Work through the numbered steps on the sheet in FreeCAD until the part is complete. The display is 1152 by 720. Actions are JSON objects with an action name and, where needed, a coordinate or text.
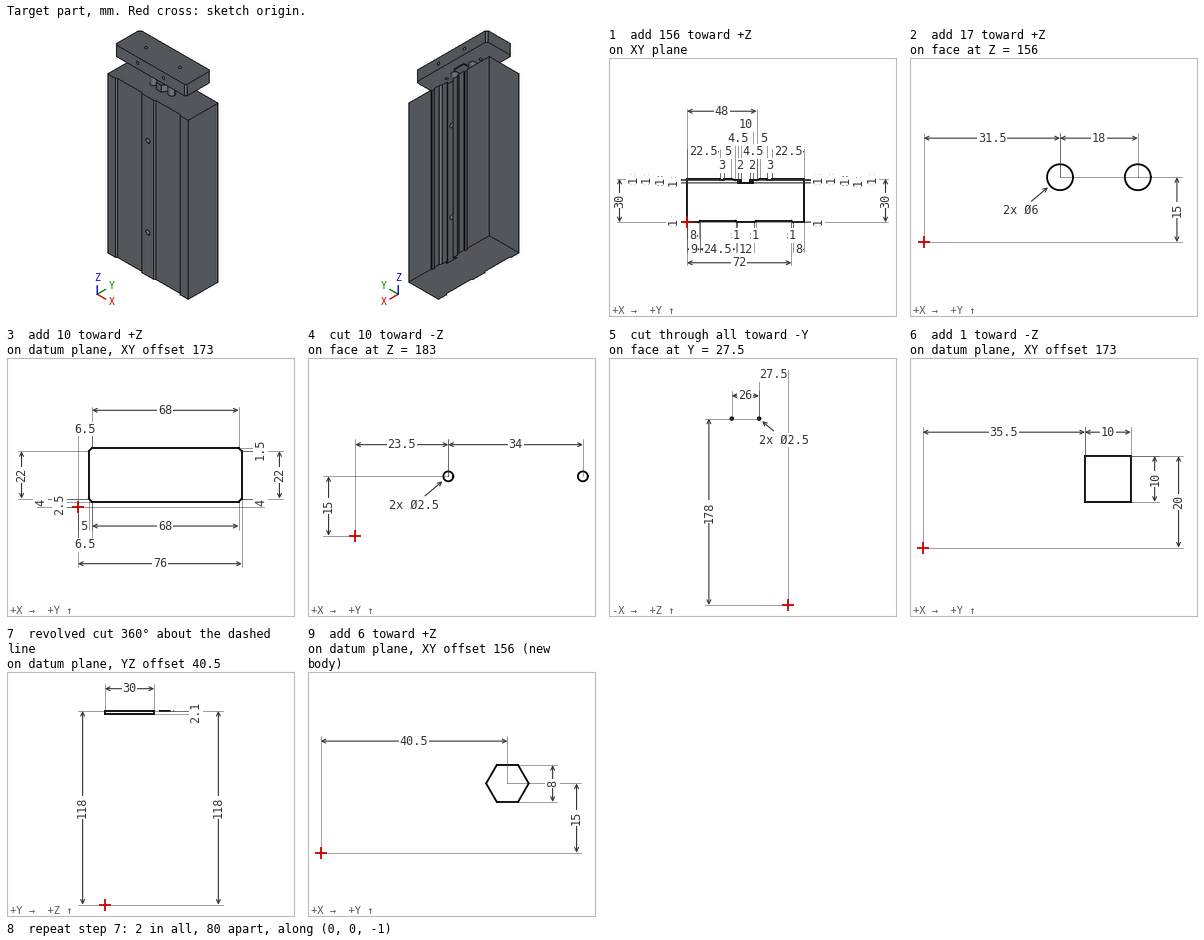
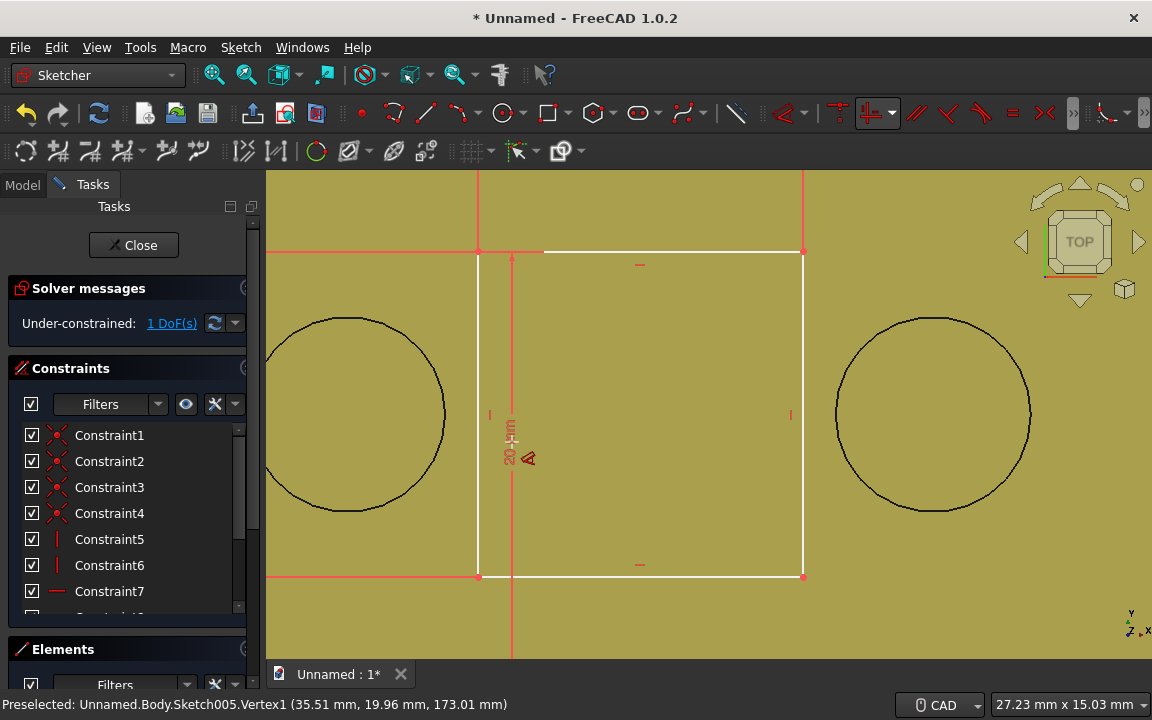
{"action": "left_click", "coordinate": [478, 252]}
{"action": "left_click", "coordinate": [386, 218]}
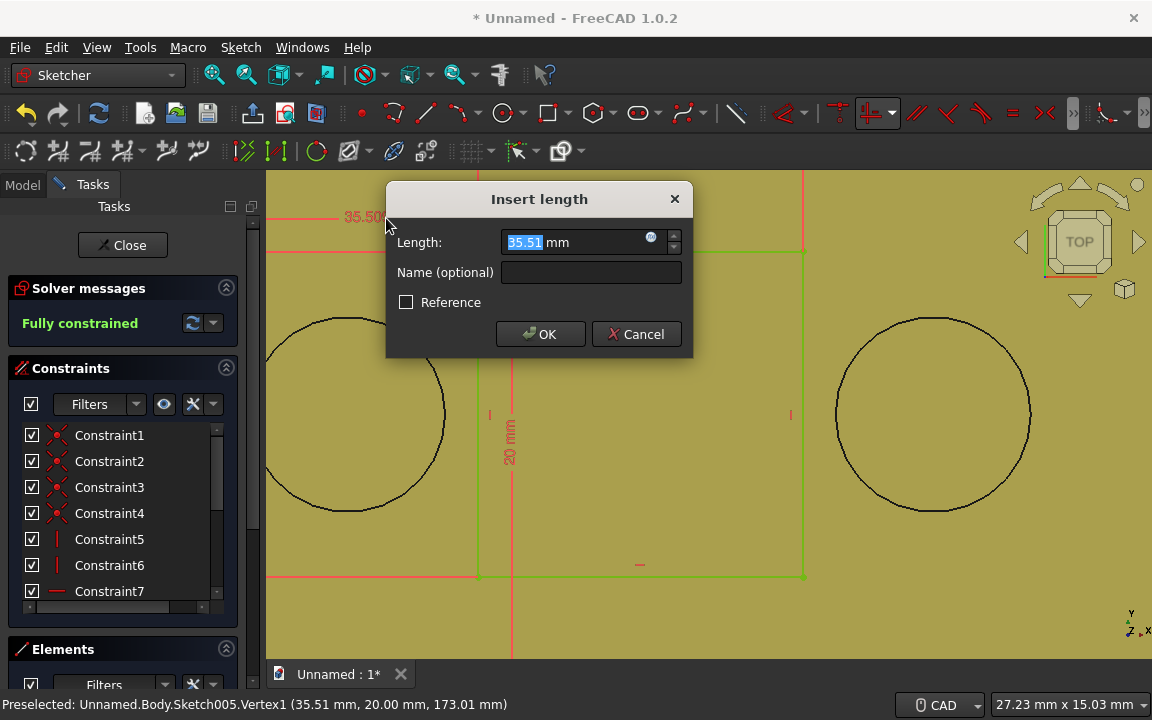
{"action": "type", "text": "35.5"}
{"action": "key", "text": "Return"}
{"action": "key", "text": "Escape"}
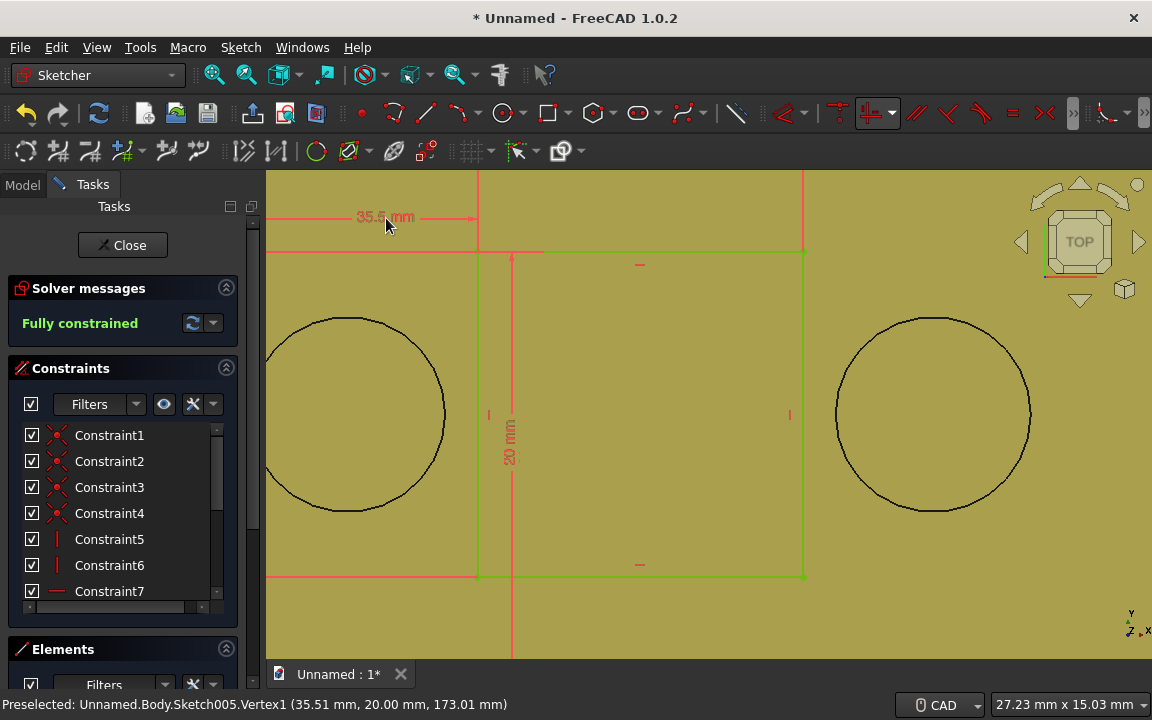
{"action": "left_click", "coordinate": [123, 245]}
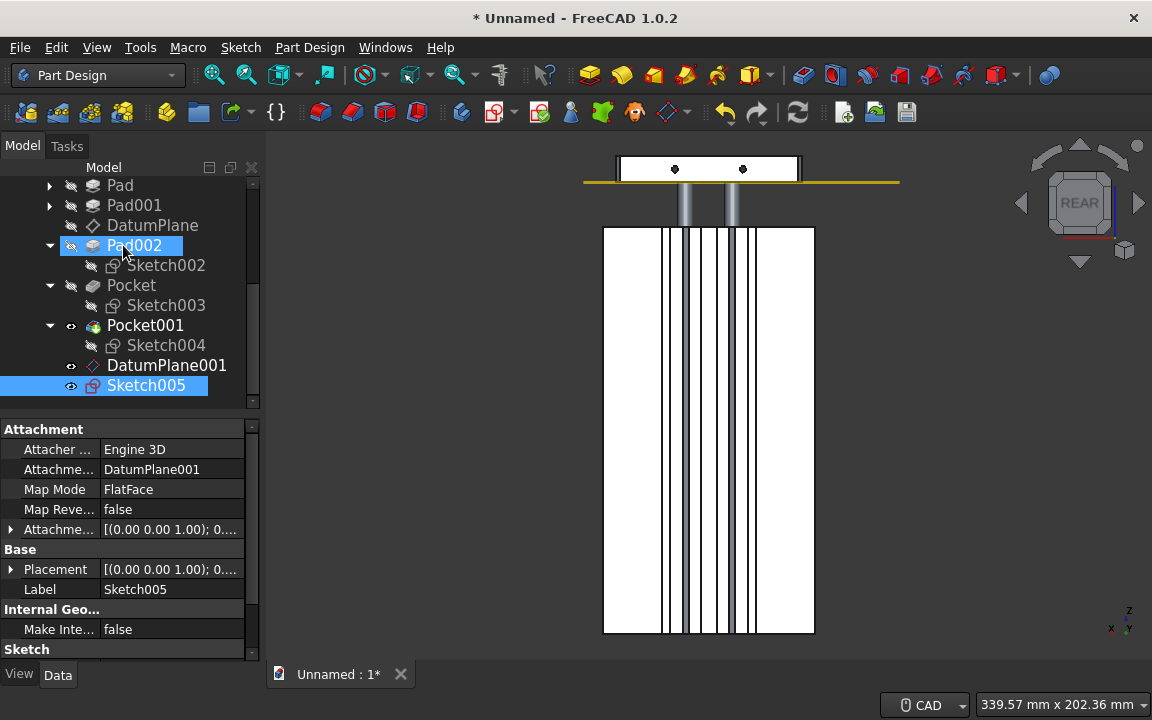
{"action": "left_click", "coordinate": [590, 76]}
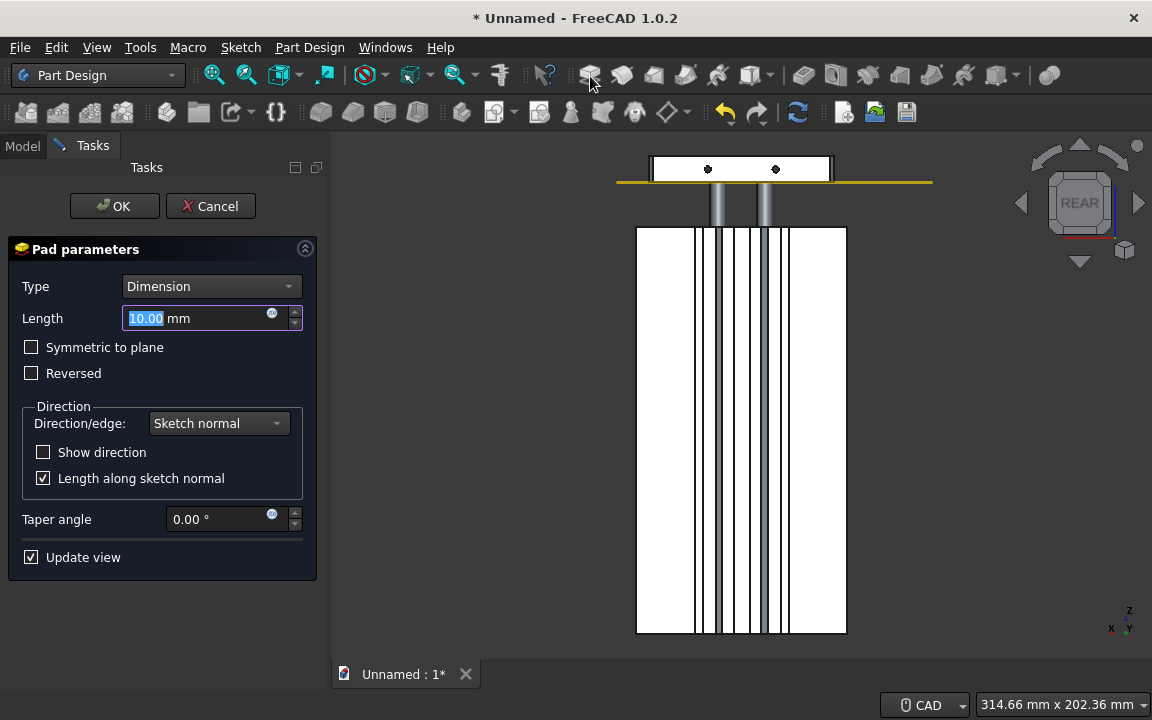
{"action": "type", "text": "1"}
{"action": "key", "text": "Tab"}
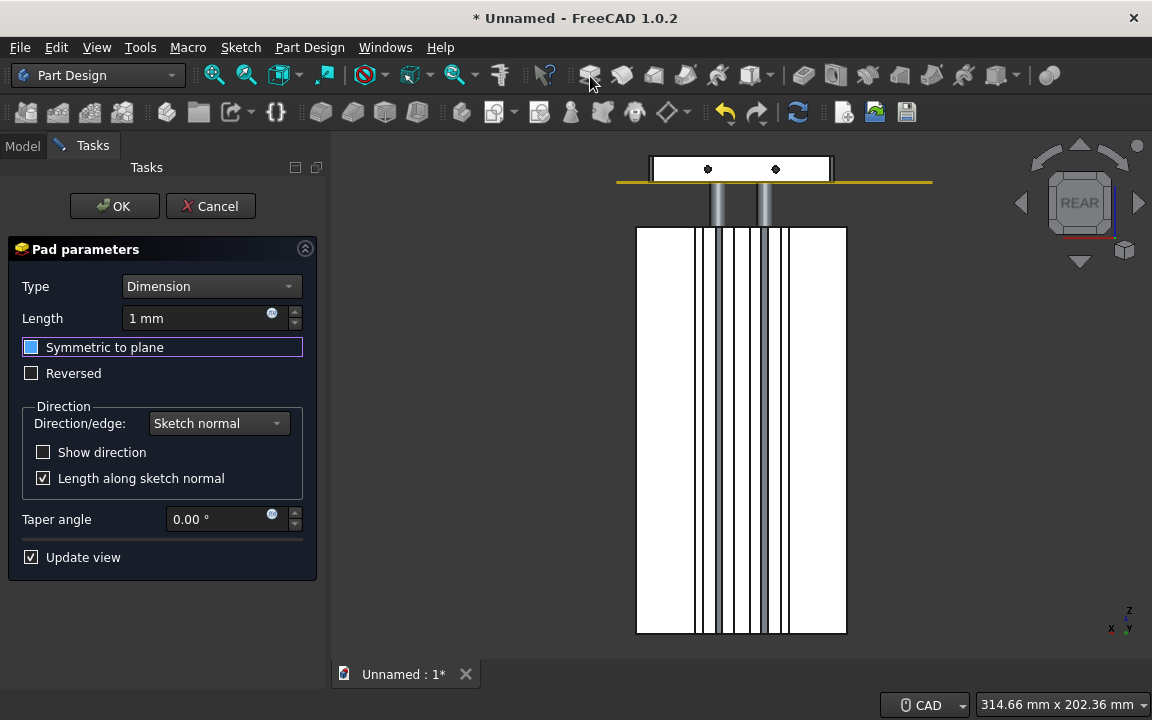
{"action": "left_click", "coordinate": [30, 373]}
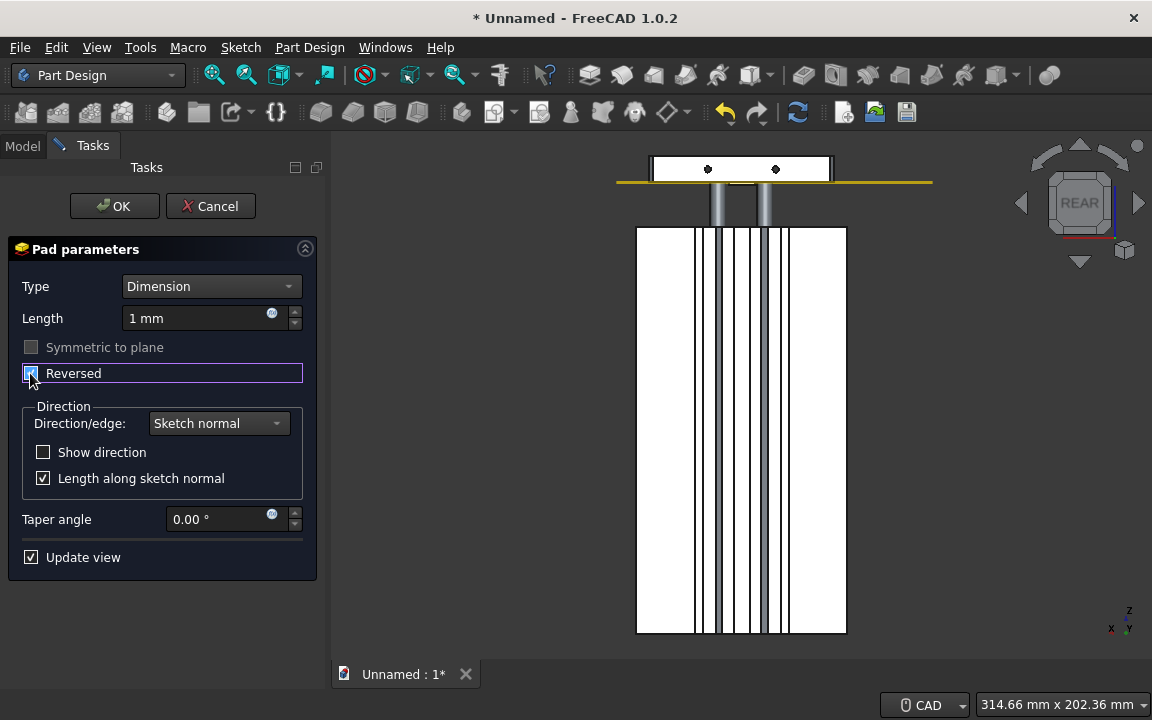
{"action": "left_click", "coordinate": [115, 206]}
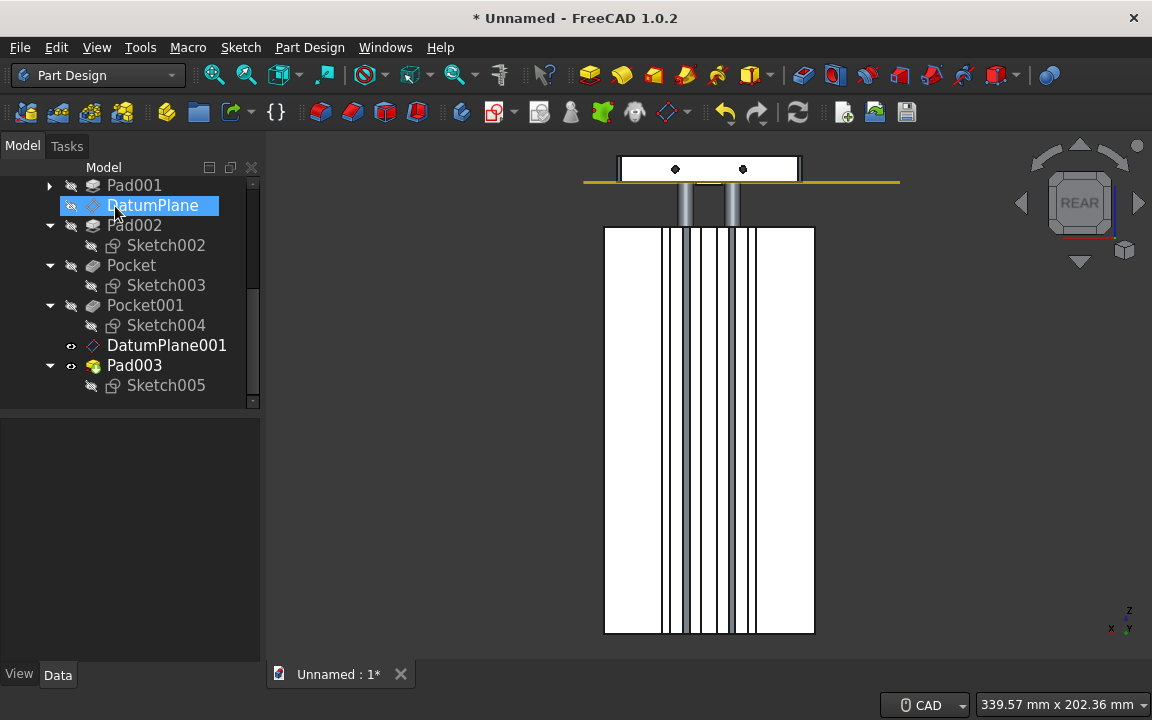
{"action": "left_click", "coordinate": [116, 346]}
{"action": "key", "text": "space"}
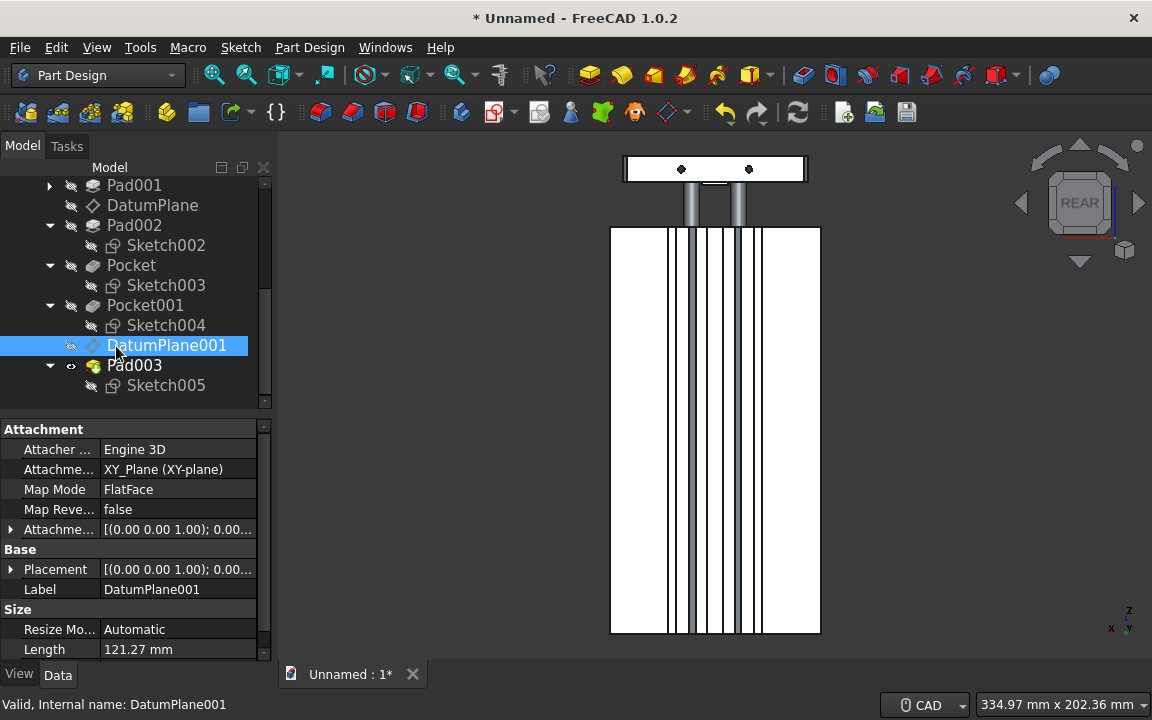
{"action": "scroll", "coordinate": [140, 281], "scroll_direction": "down", "scroll_amount": 3}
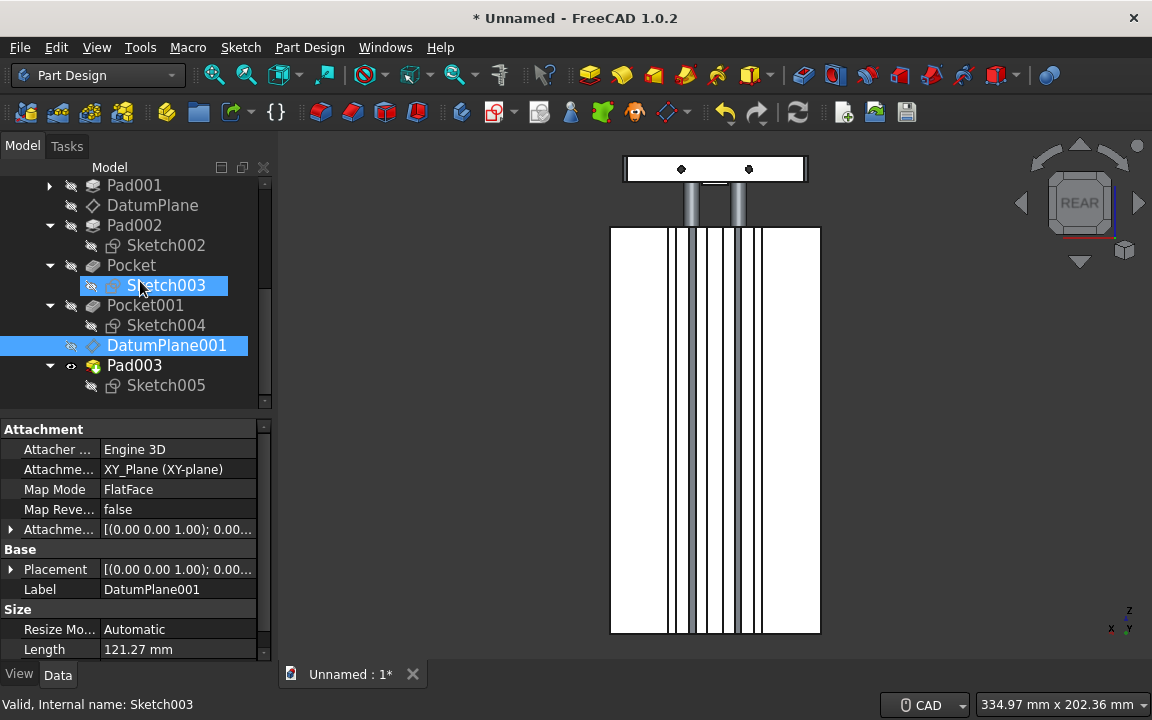
{"action": "scroll", "coordinate": [140, 281], "scroll_direction": "up", "scroll_amount": 15}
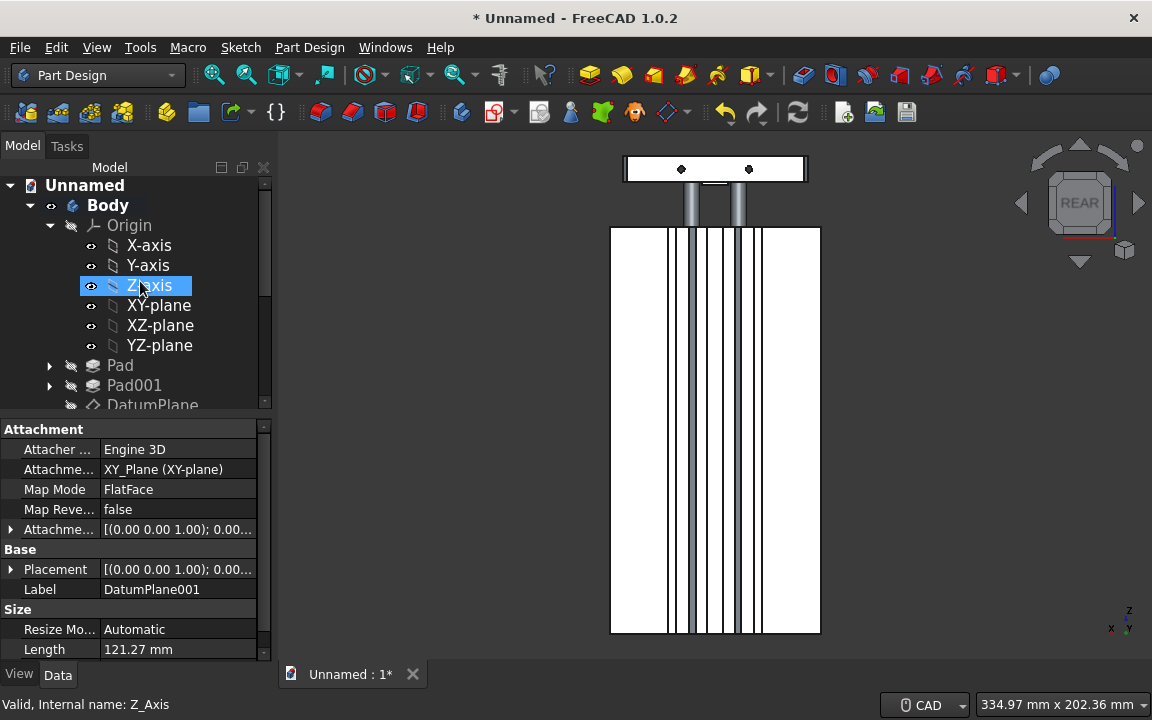
{"action": "left_click", "coordinate": [136, 346]}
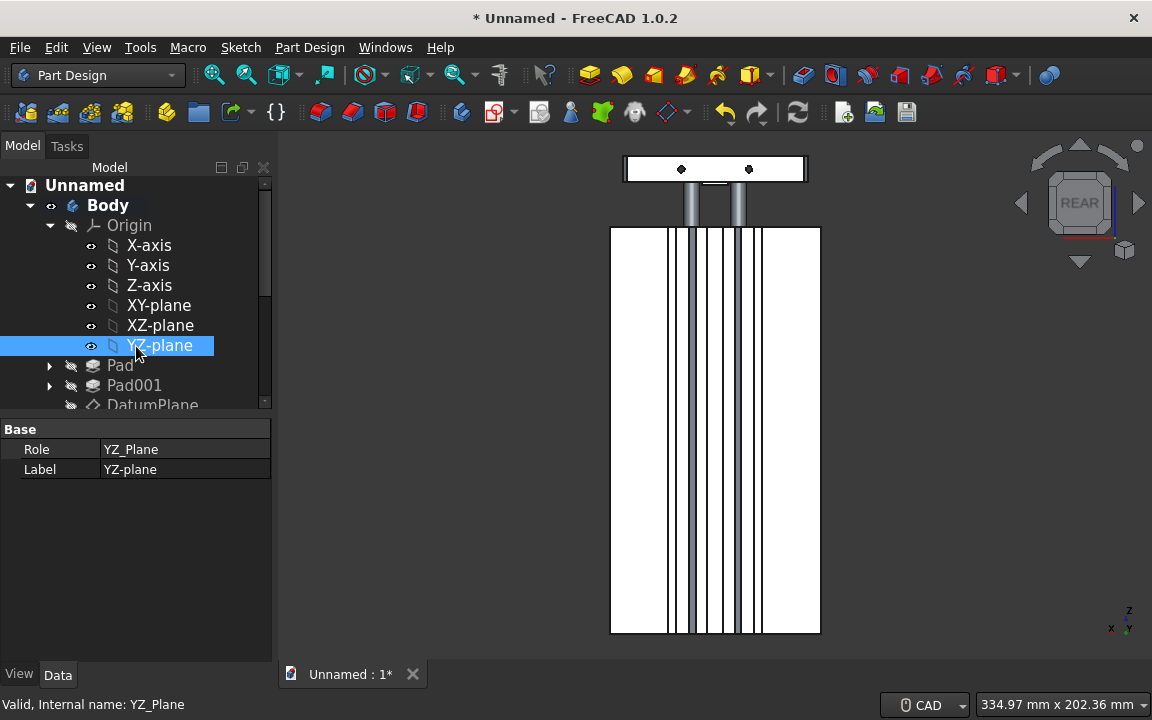
{"action": "left_click", "coordinate": [668, 112]}